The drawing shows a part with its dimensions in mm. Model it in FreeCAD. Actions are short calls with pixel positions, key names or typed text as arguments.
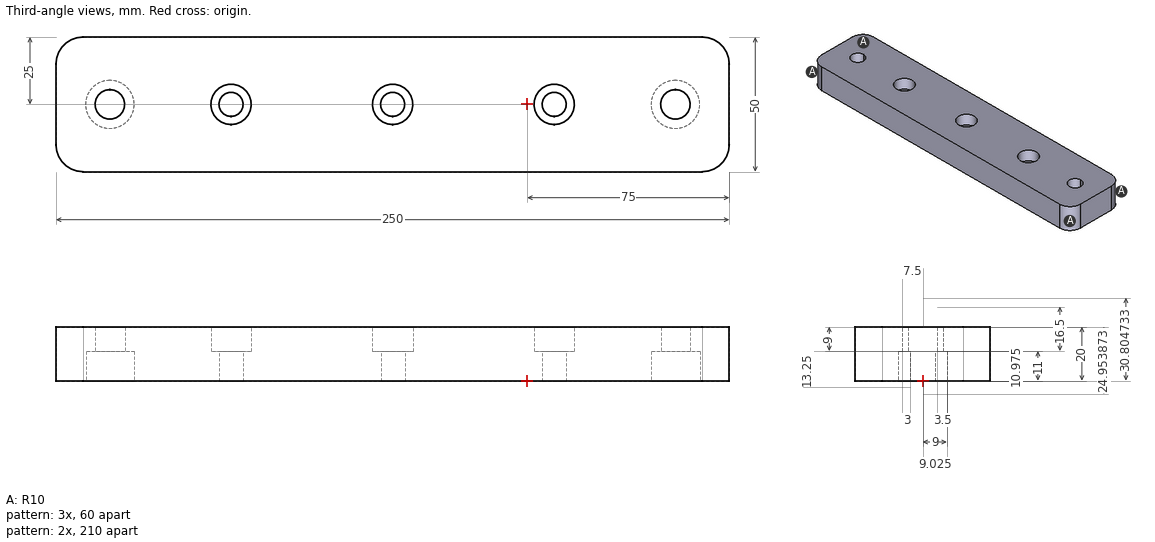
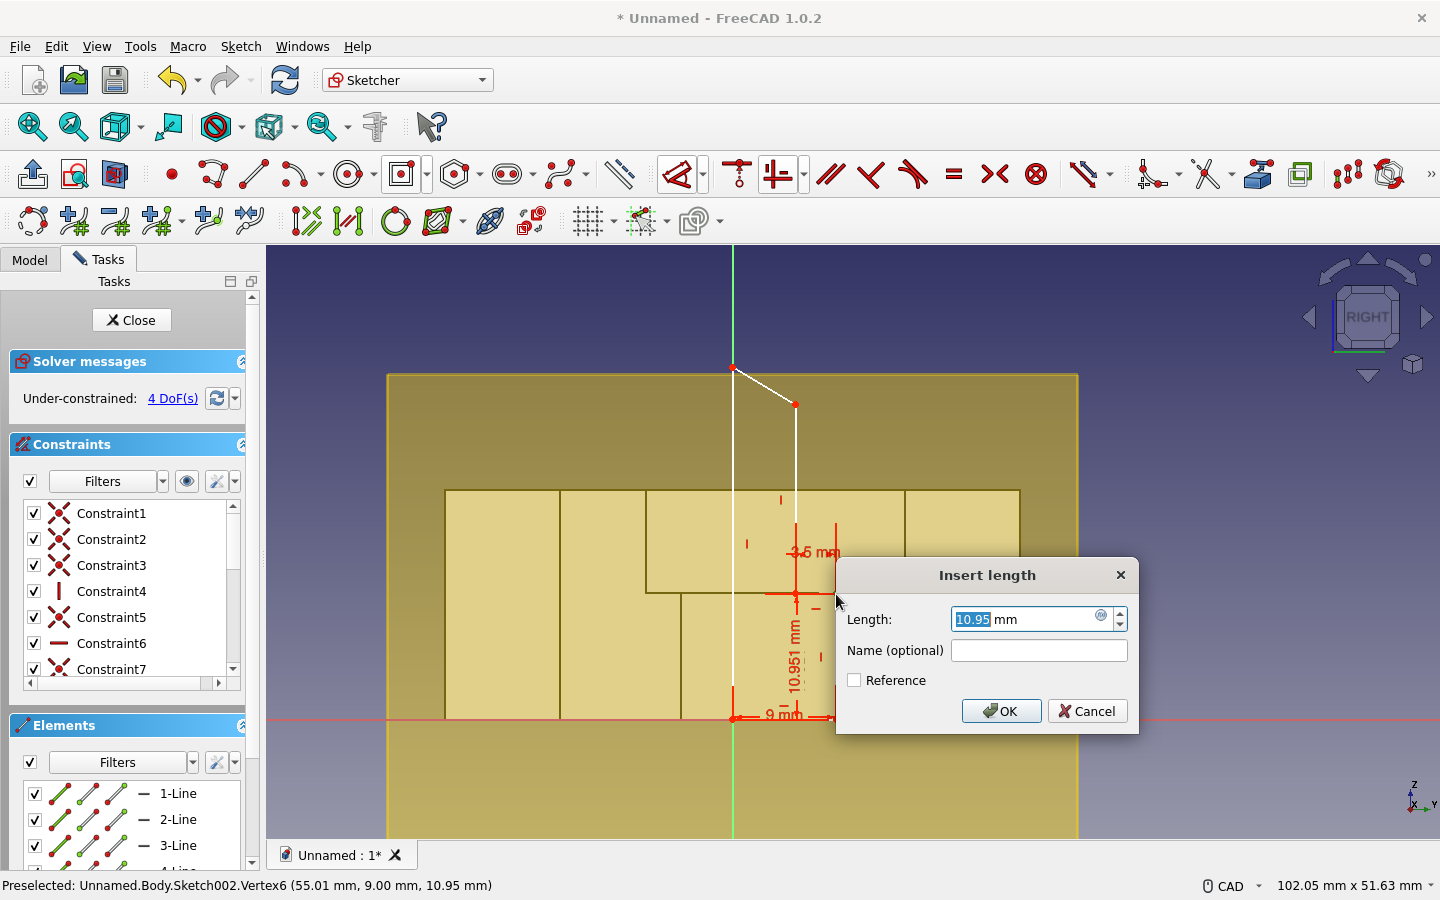
text(11)
key(Return)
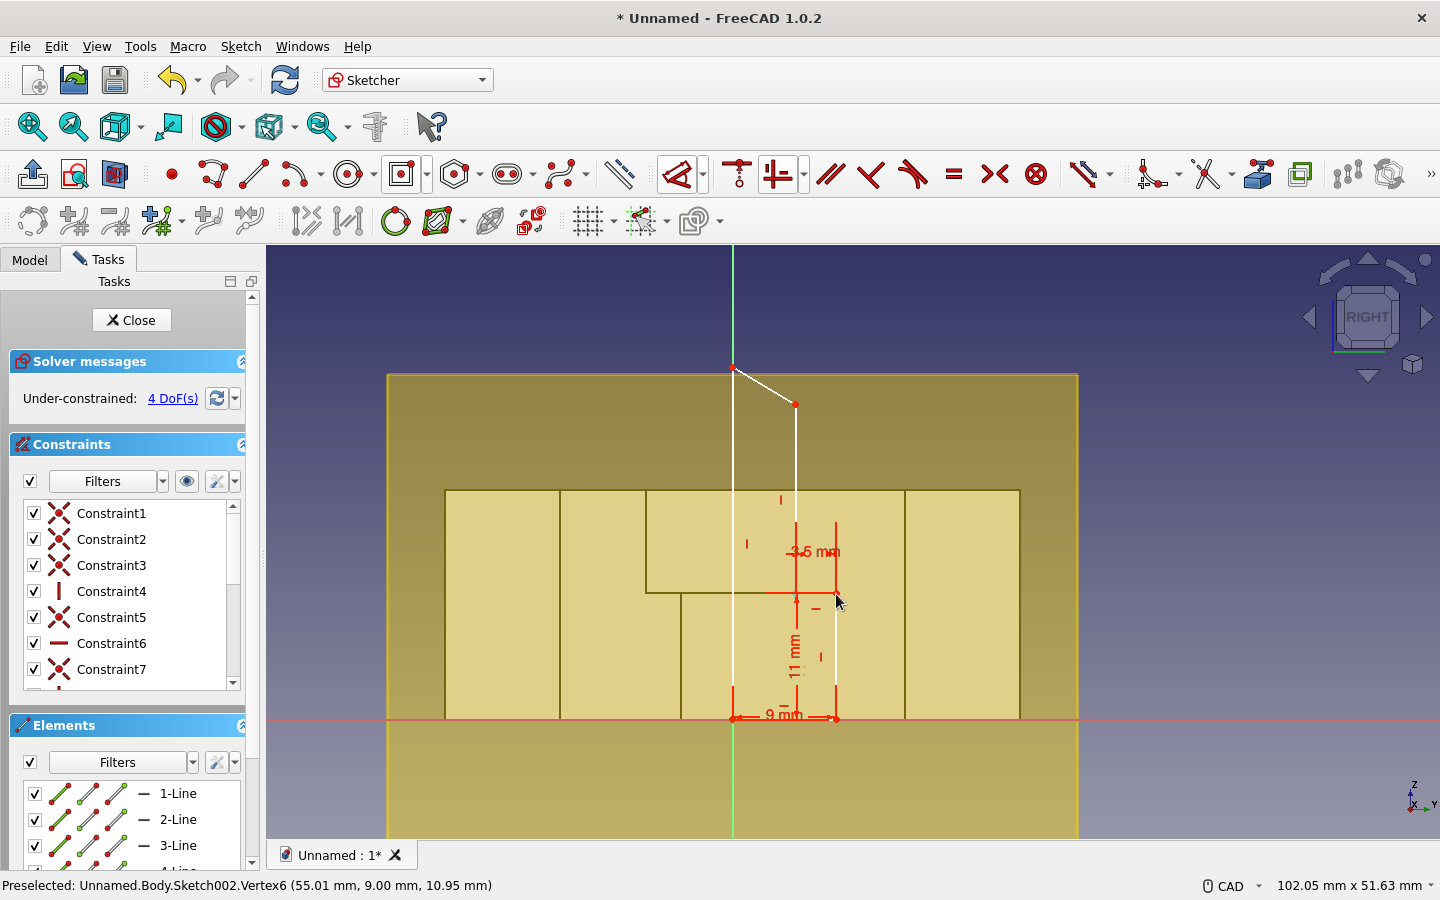
click(796, 537)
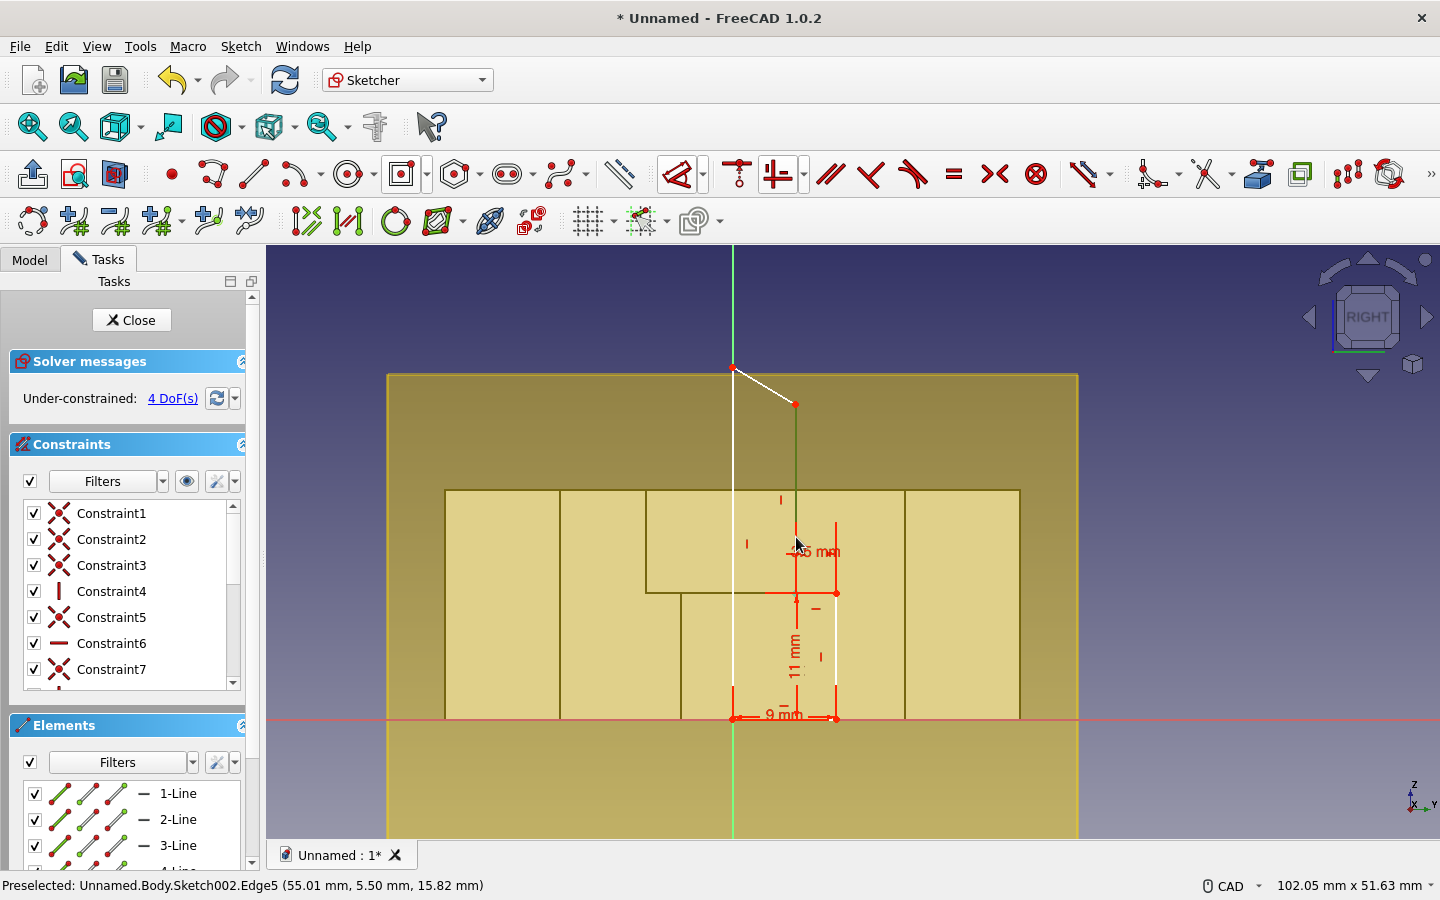
key(i)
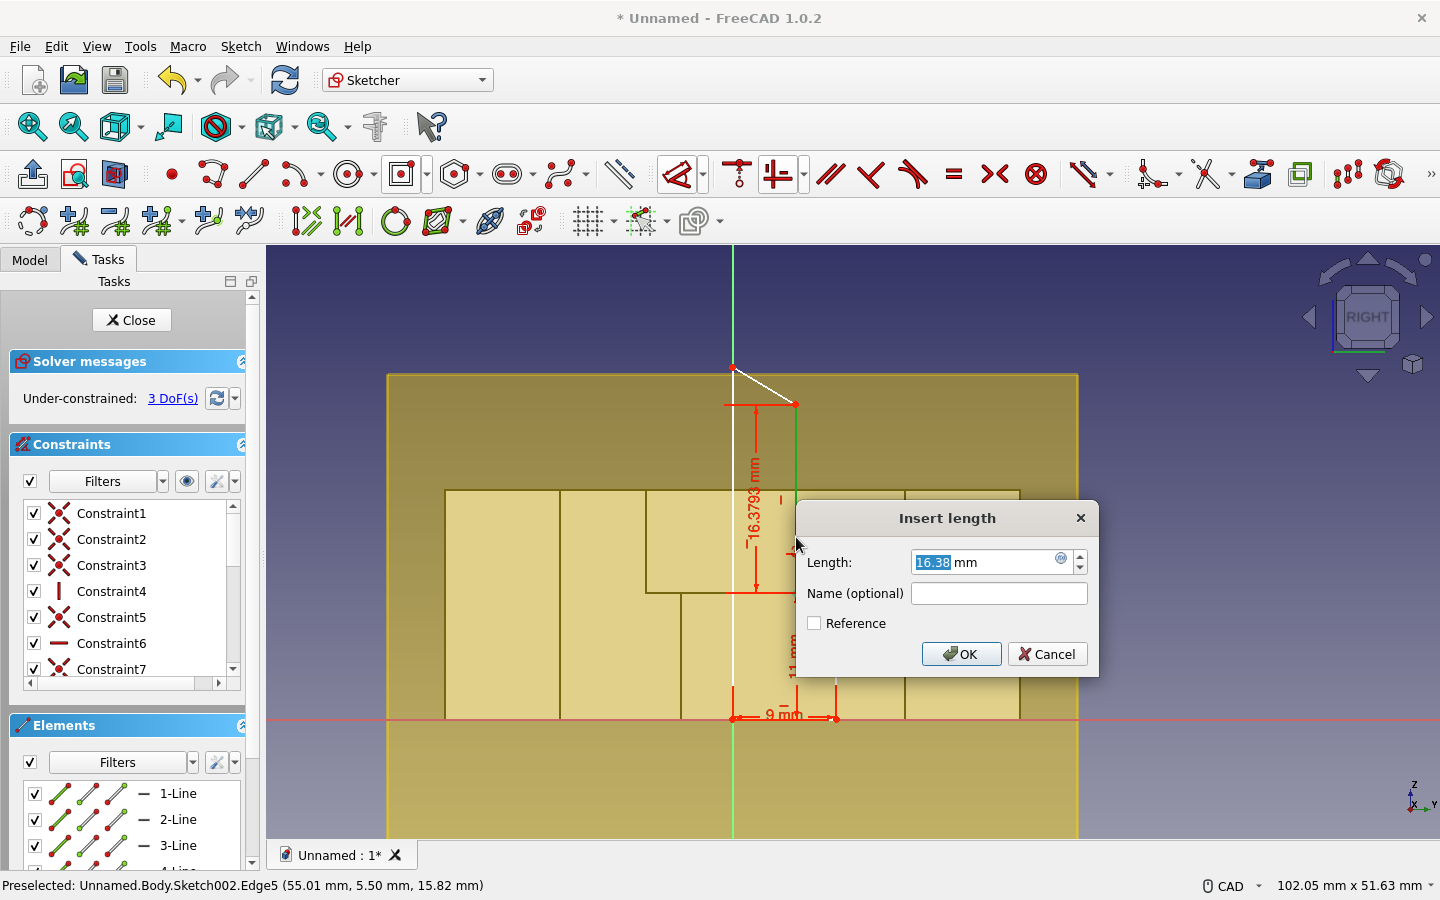
text(16.5)
key(Return)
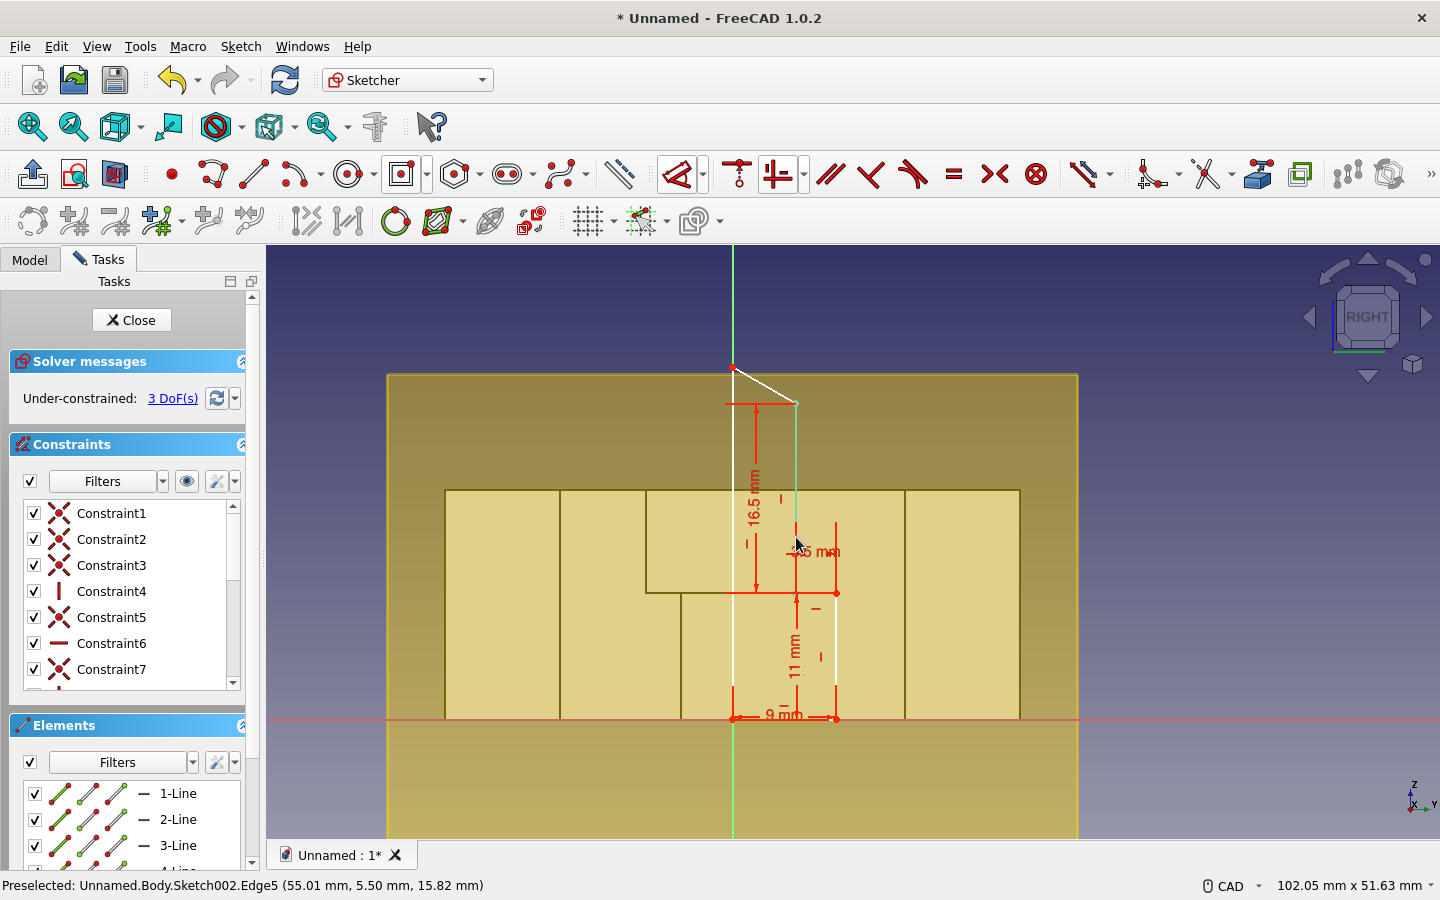
click(764, 720)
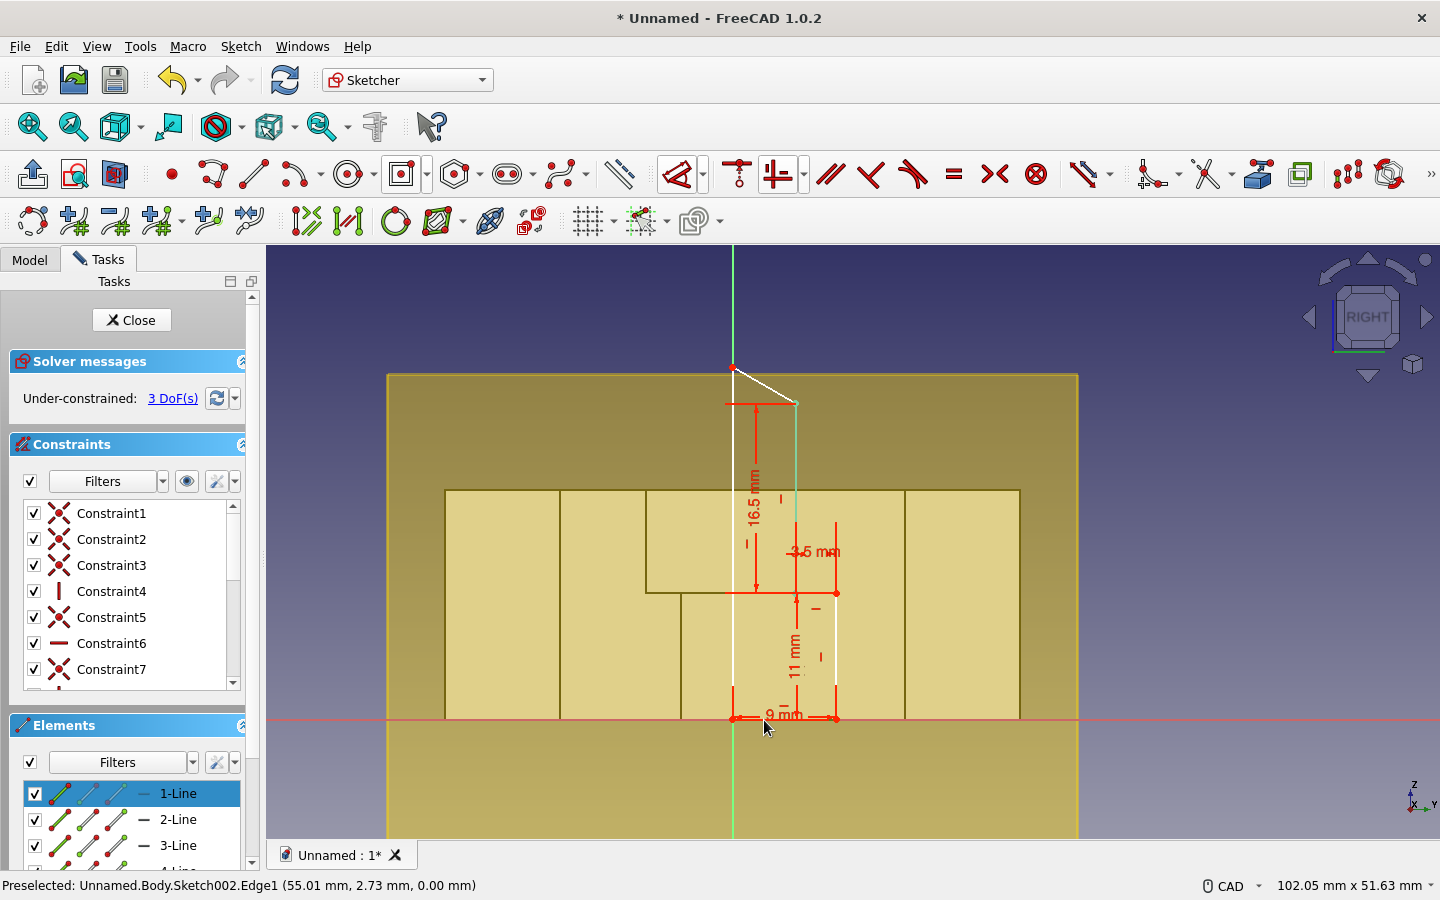
key(l)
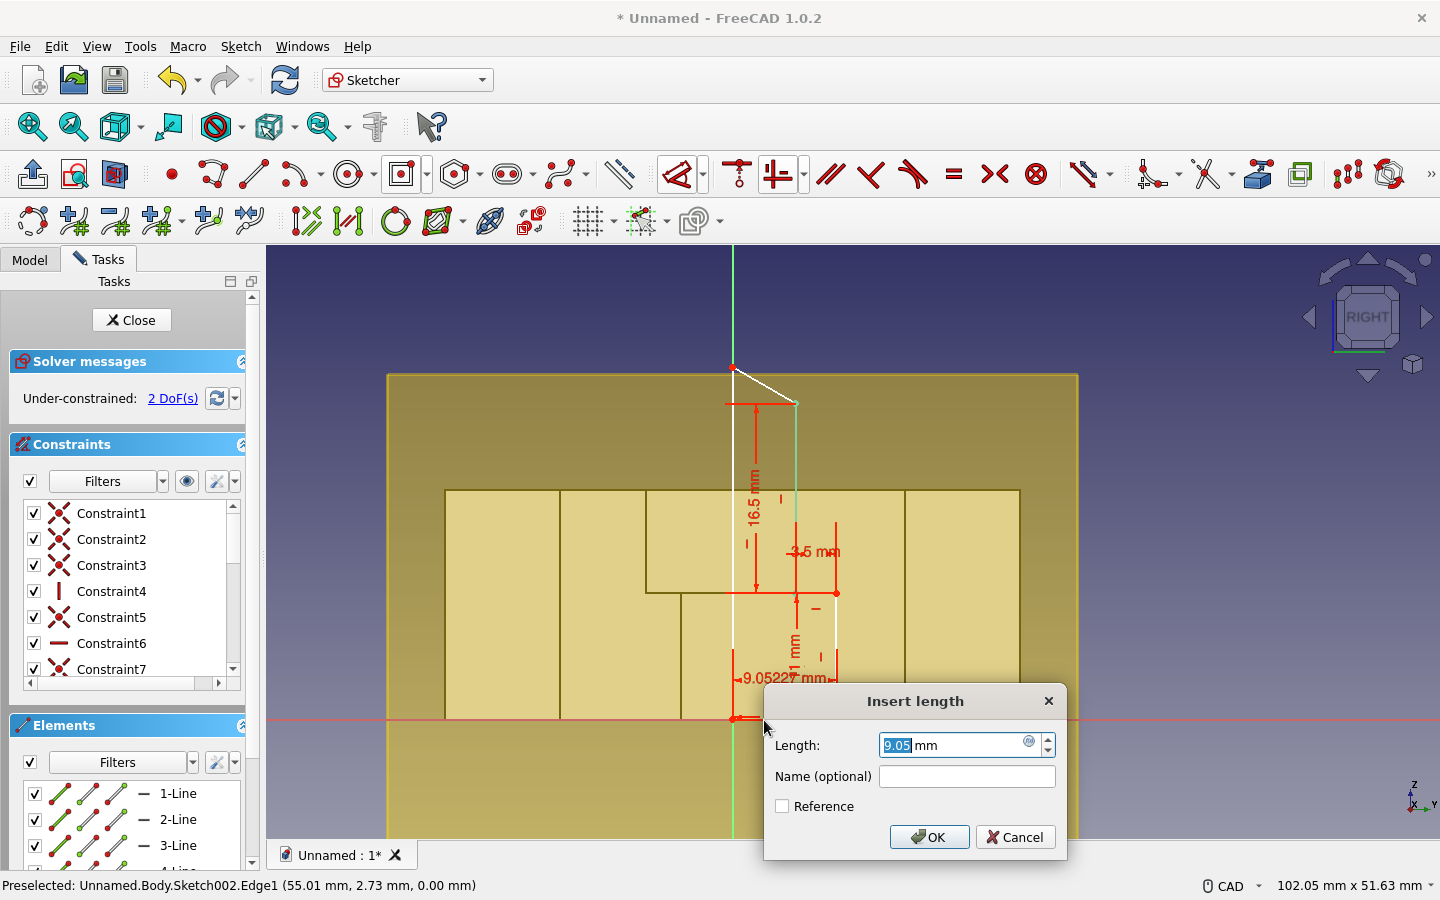
text(9.025)
key(Return)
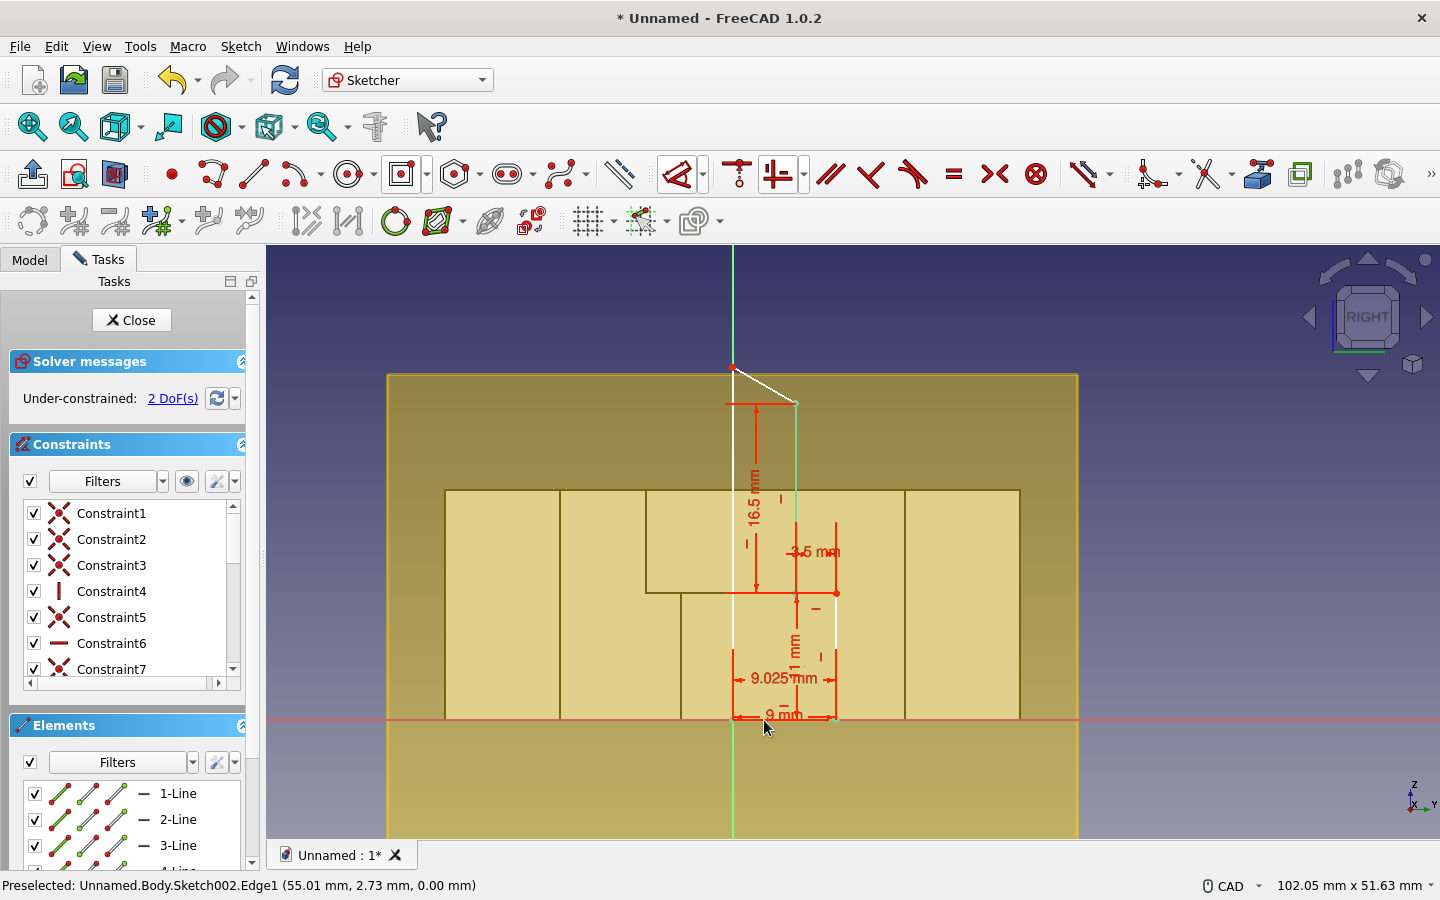
click(836, 682)